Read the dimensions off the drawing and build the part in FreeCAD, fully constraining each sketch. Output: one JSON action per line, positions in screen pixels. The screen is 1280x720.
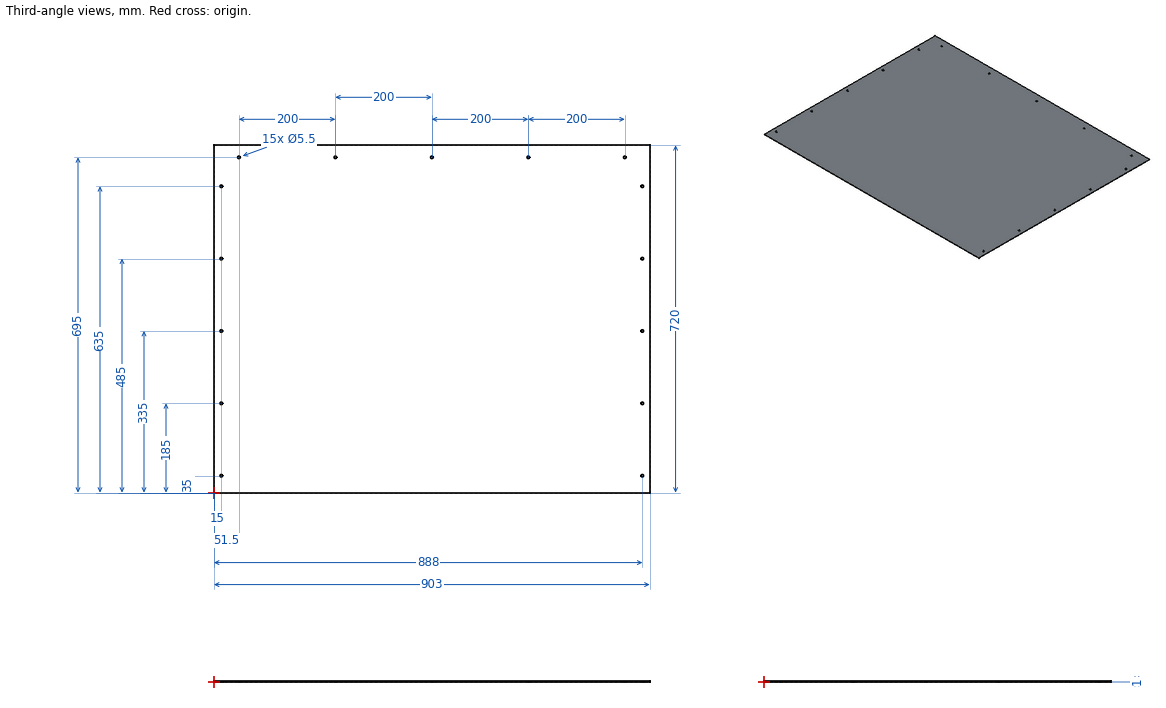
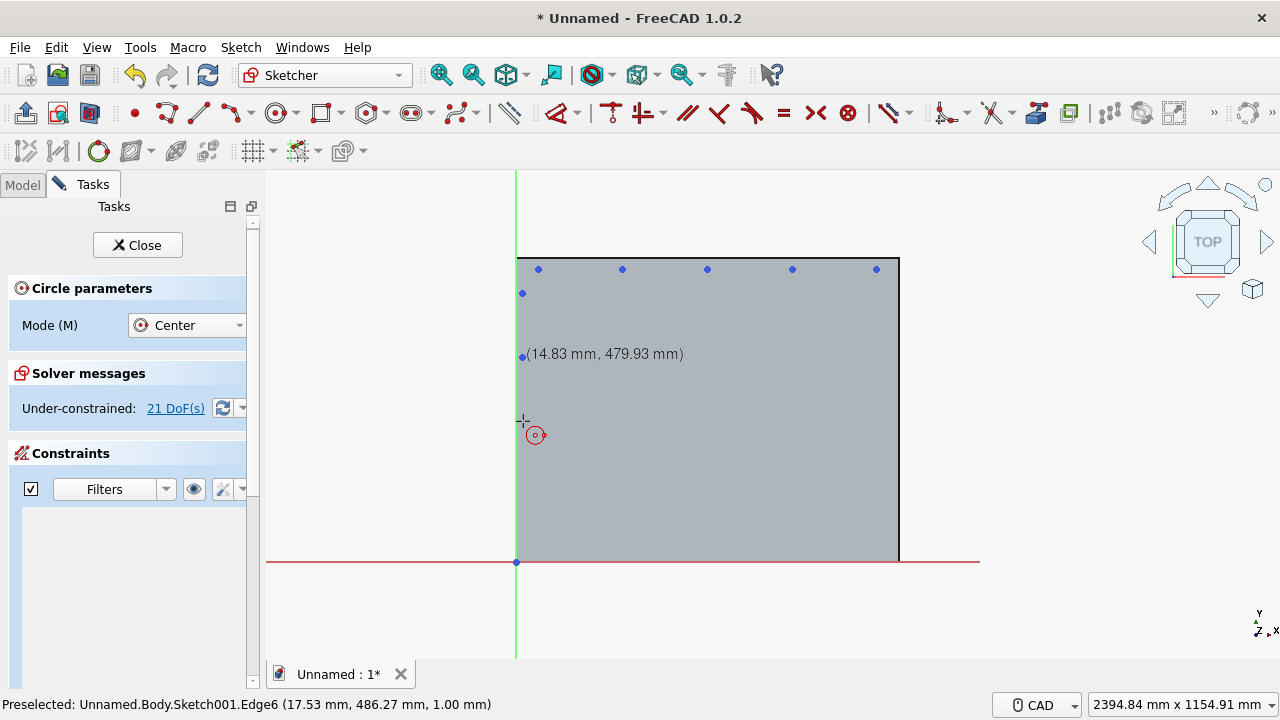
{"action": "scroll", "coordinate": [523, 421], "scroll_direction": "up", "scroll_amount": 5}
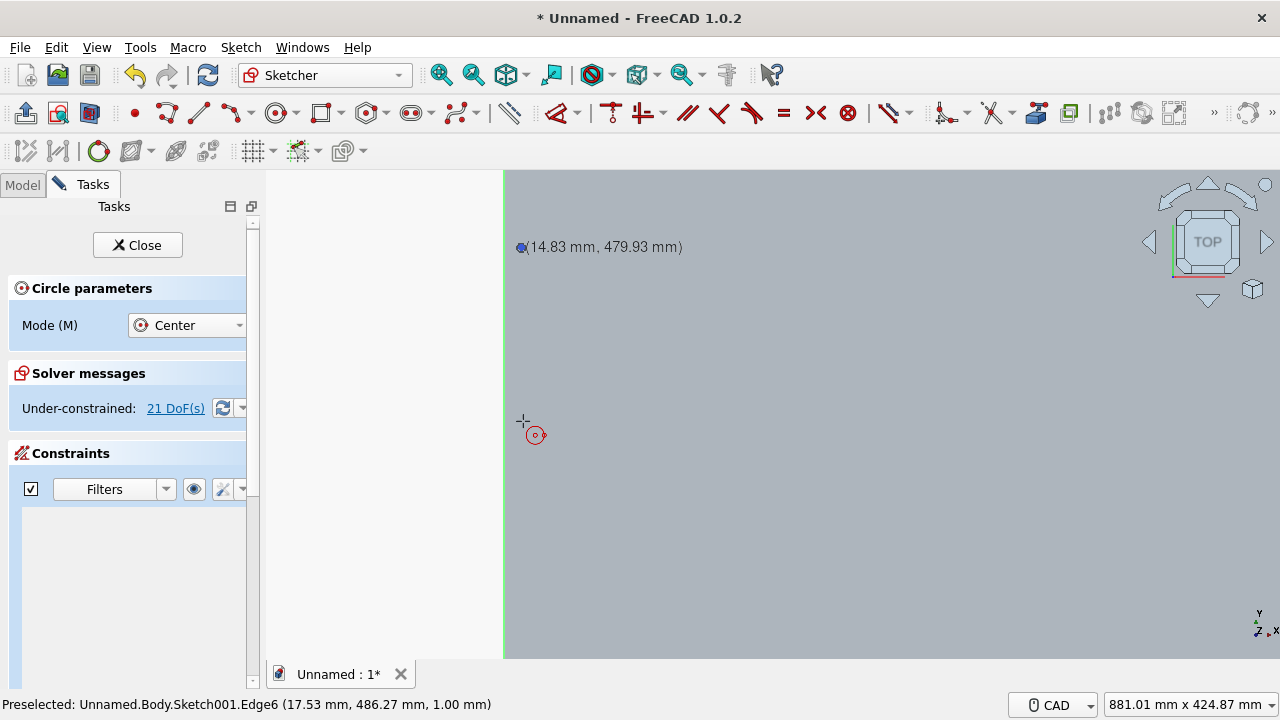
{"action": "left_click", "coordinate": [521, 419]}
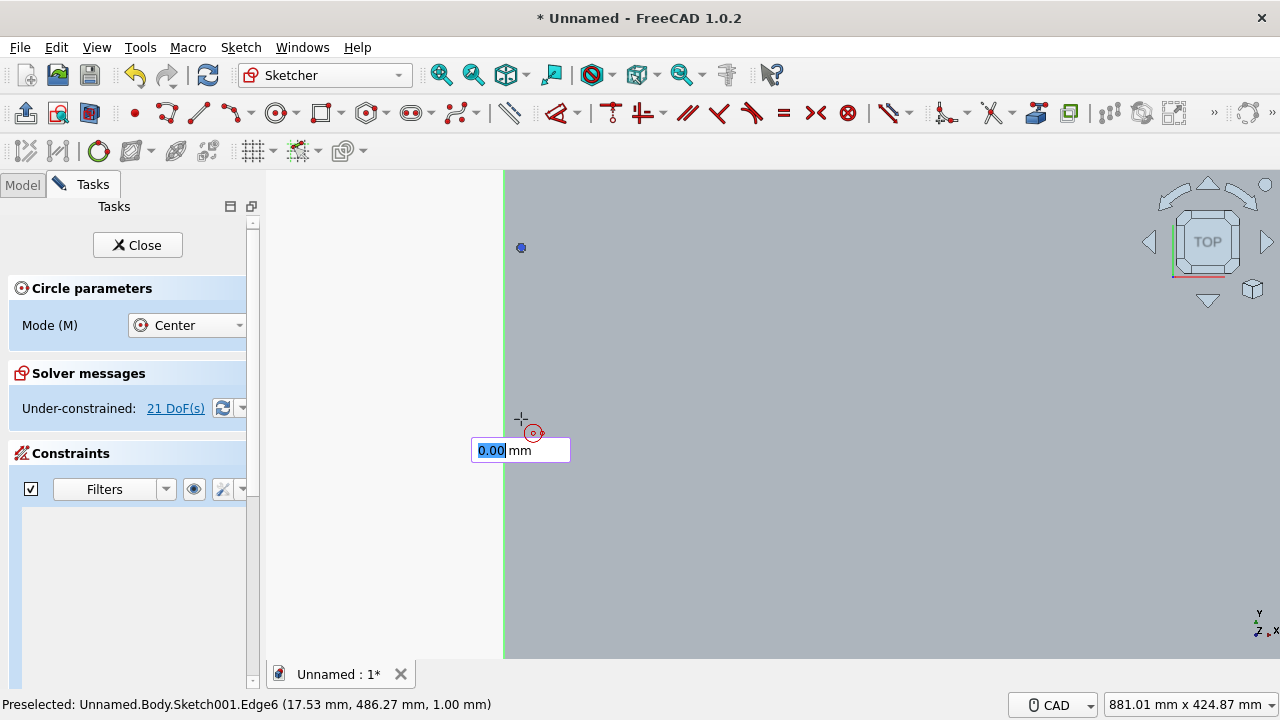
{"action": "scroll", "coordinate": [524, 417], "scroll_direction": "up", "scroll_amount": 9}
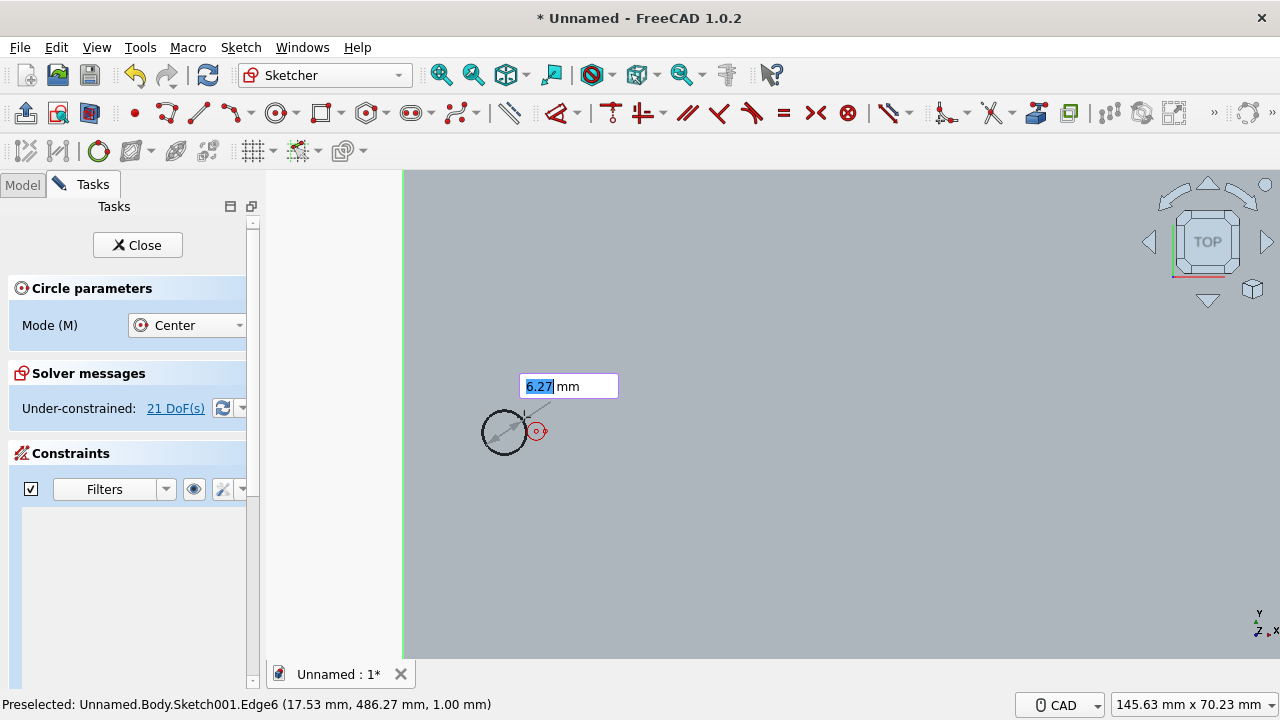
{"action": "left_click", "coordinate": [520, 413]}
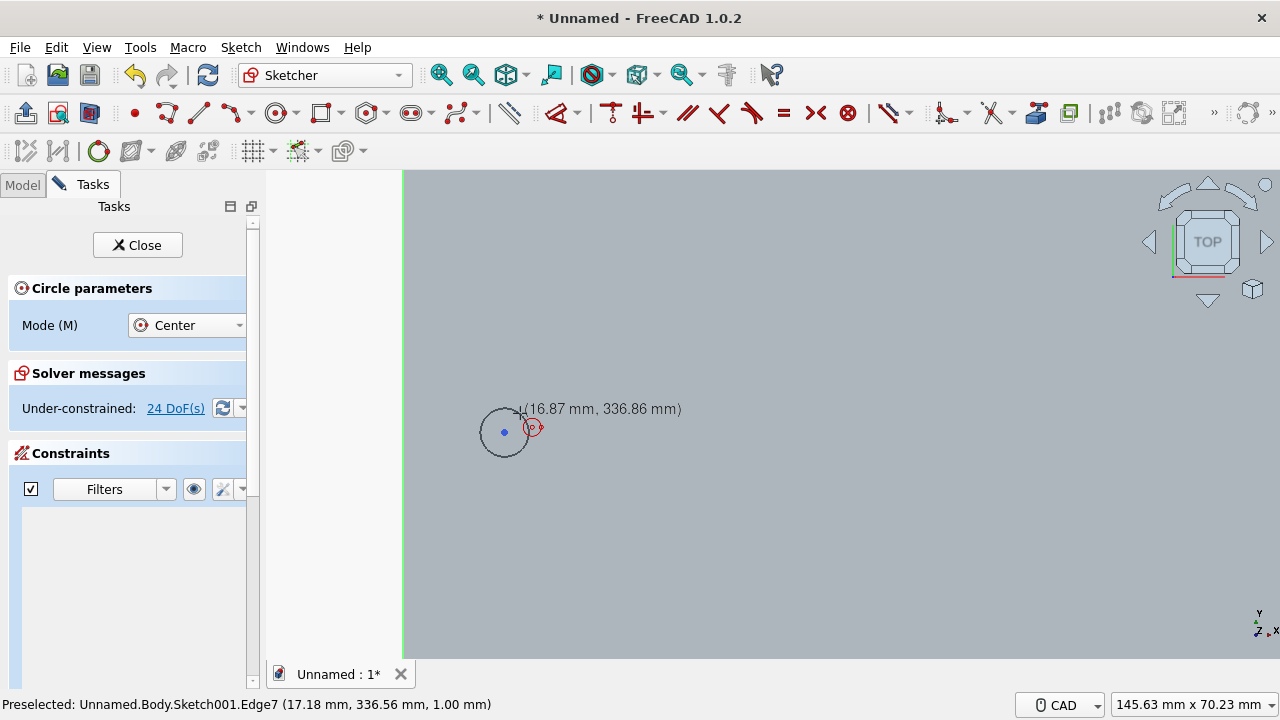
{"action": "scroll", "coordinate": [523, 420], "scroll_direction": "down", "scroll_amount": 14}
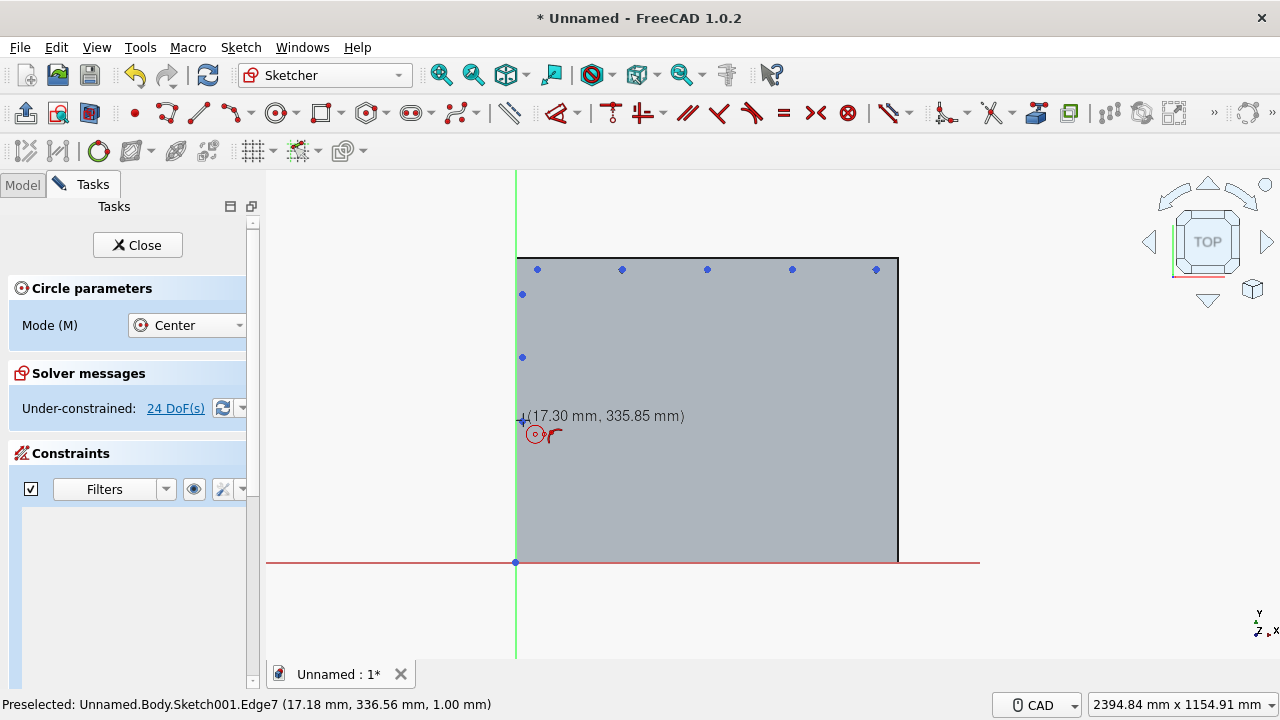
{"action": "scroll", "coordinate": [522, 484], "scroll_direction": "up", "scroll_amount": 15}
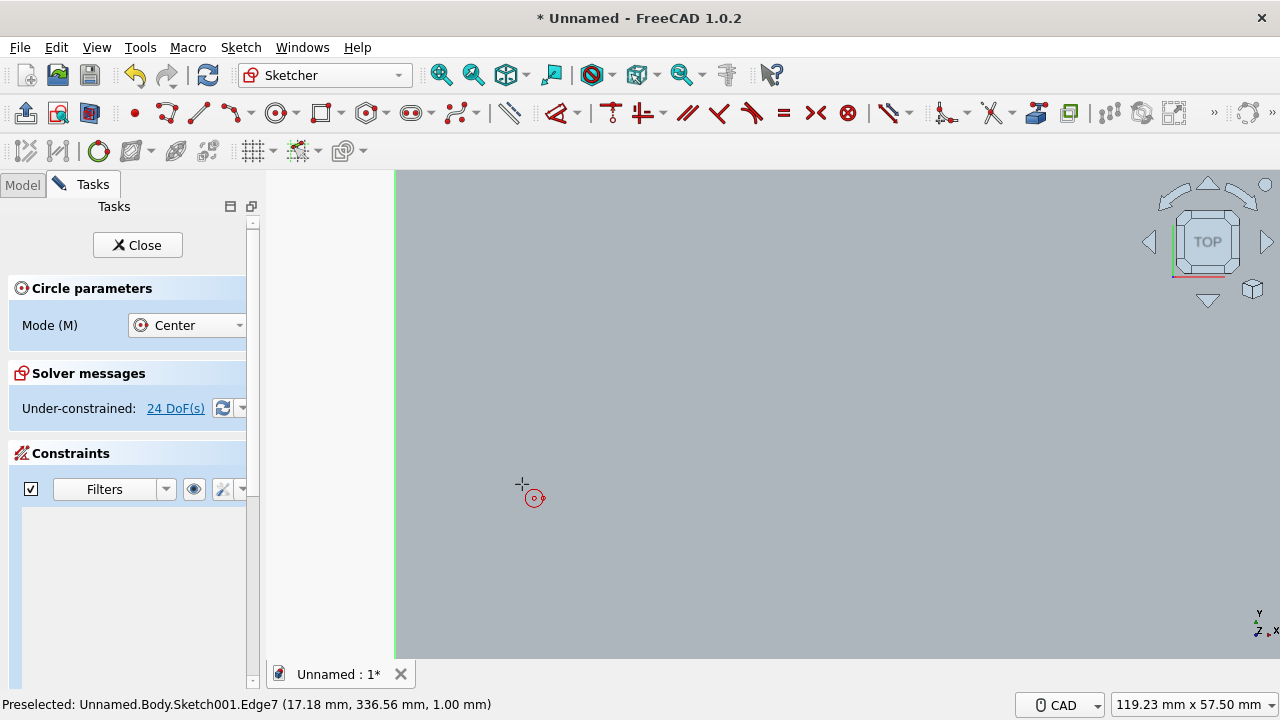
{"action": "scroll", "coordinate": [522, 484], "scroll_direction": "down", "scroll_amount": 15}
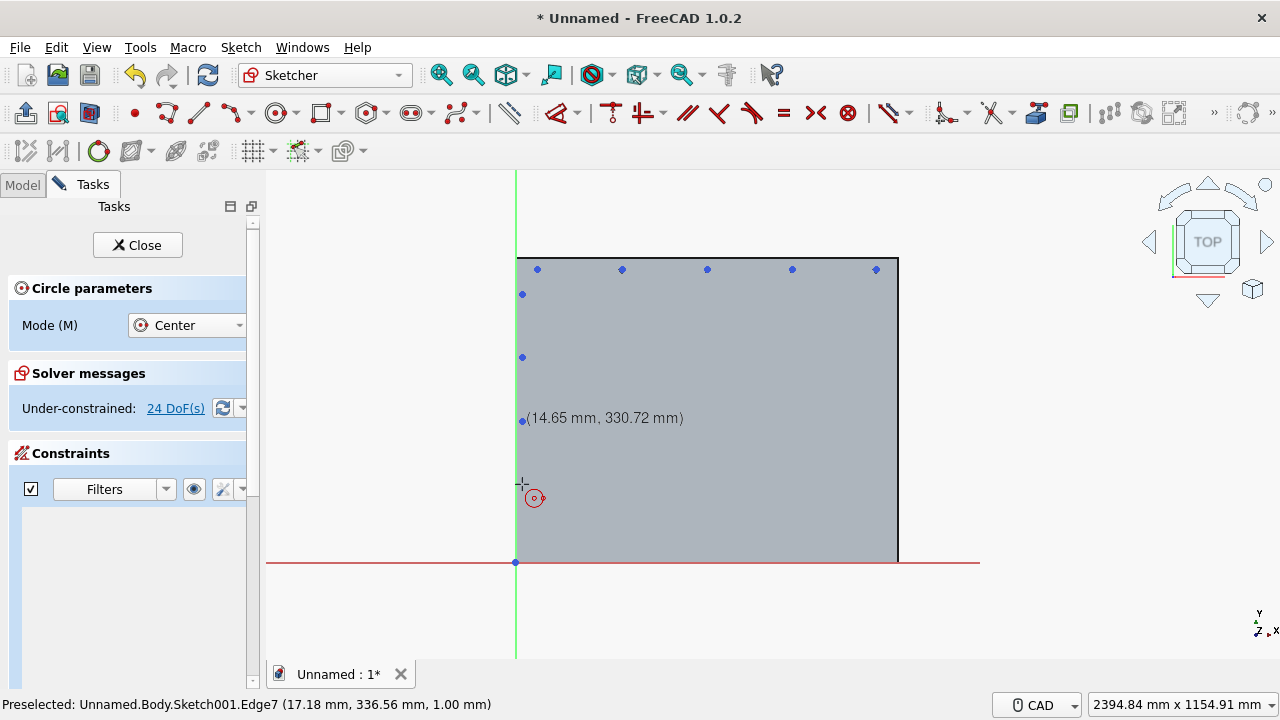
{"action": "scroll", "coordinate": [522, 484], "scroll_direction": "up", "scroll_amount": 5}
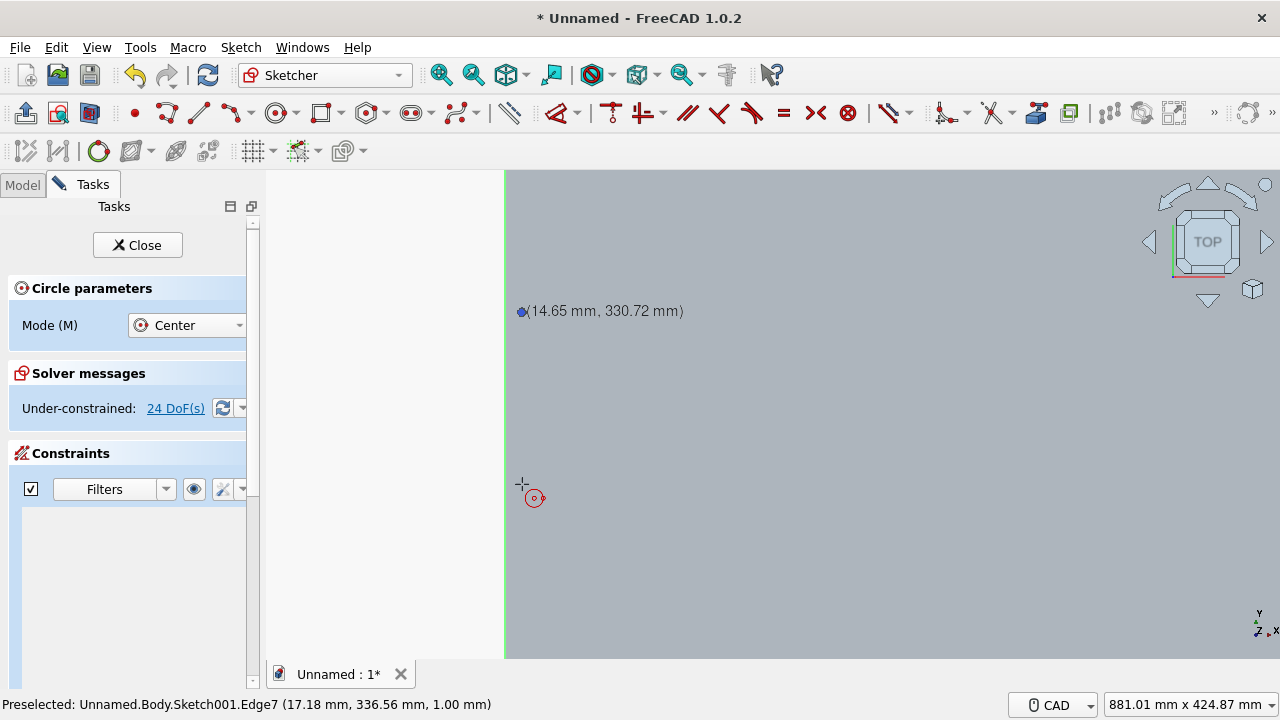
{"action": "left_click", "coordinate": [522, 484]}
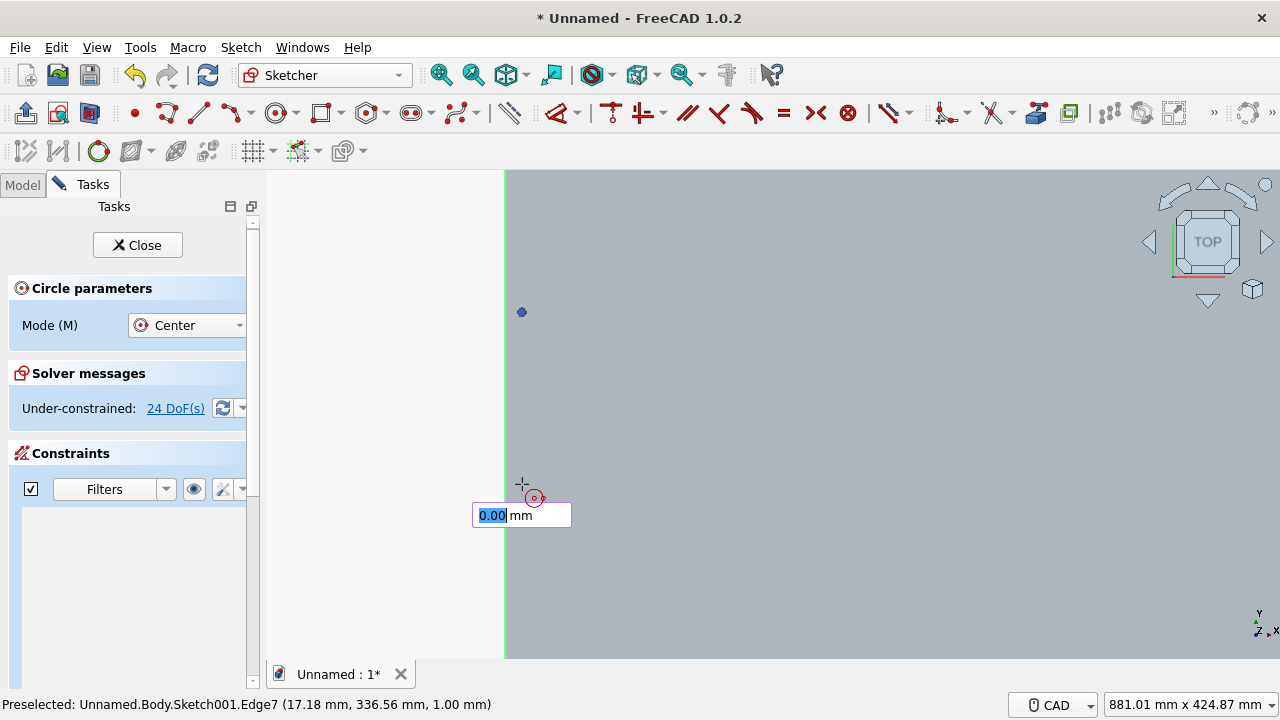
{"action": "scroll", "coordinate": [525, 482], "scroll_direction": "up", "scroll_amount": 9}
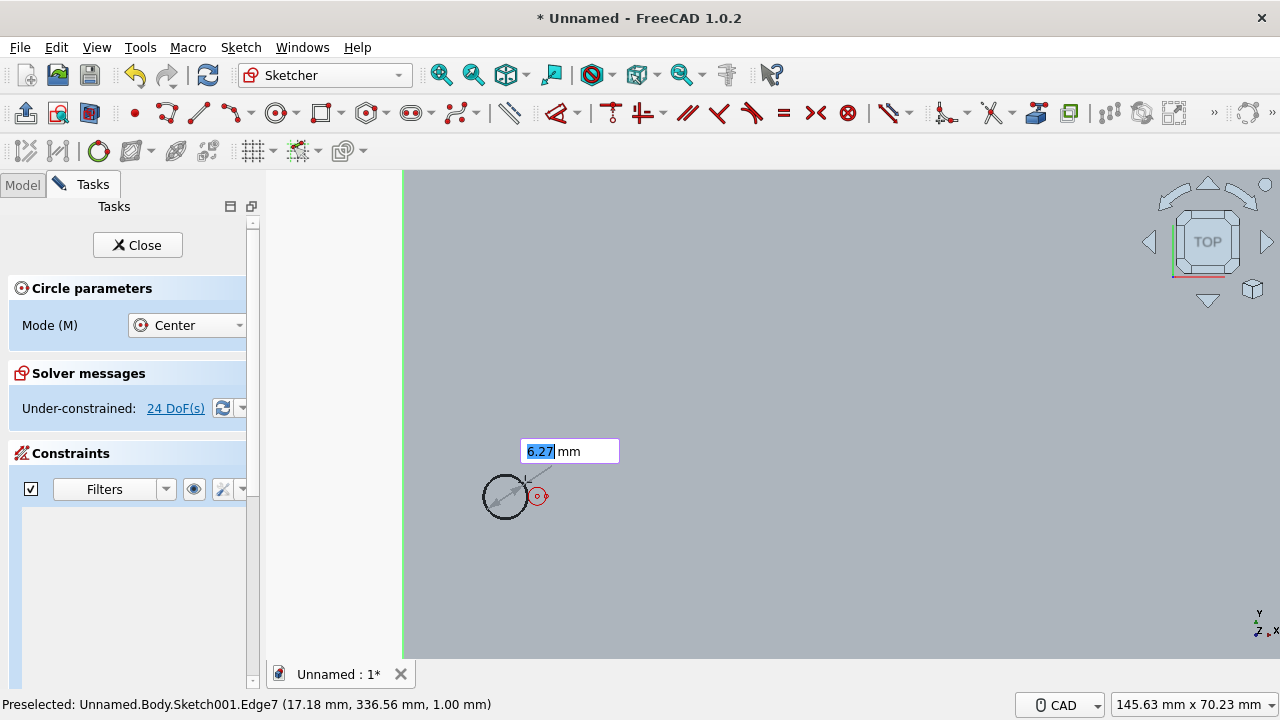
{"action": "left_click", "coordinate": [521, 477]}